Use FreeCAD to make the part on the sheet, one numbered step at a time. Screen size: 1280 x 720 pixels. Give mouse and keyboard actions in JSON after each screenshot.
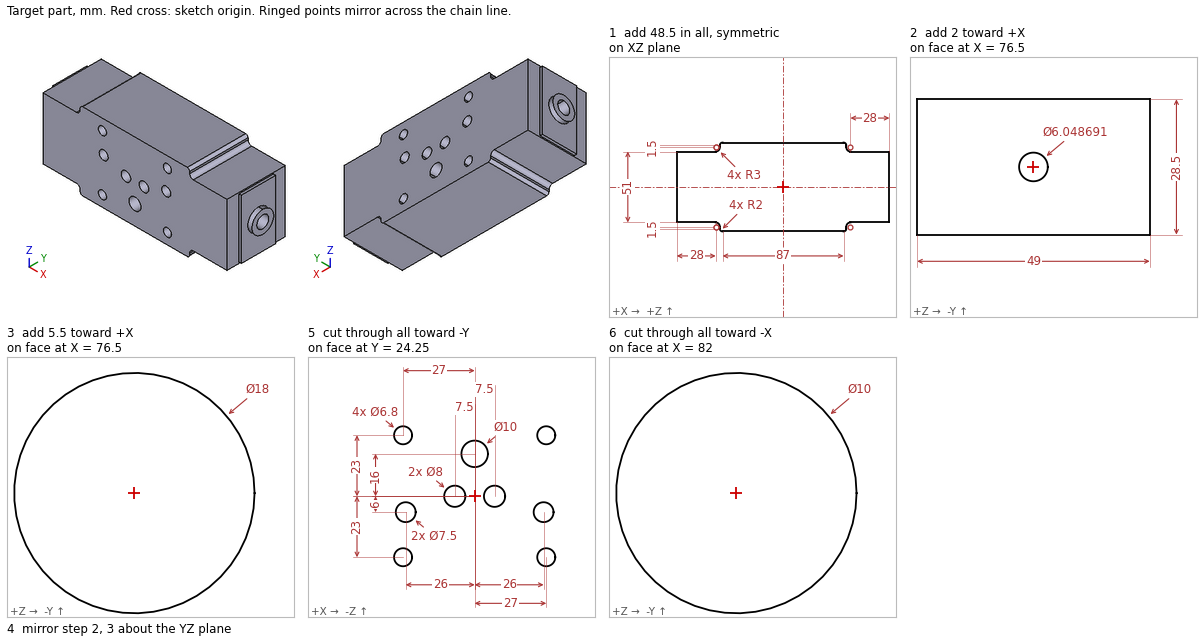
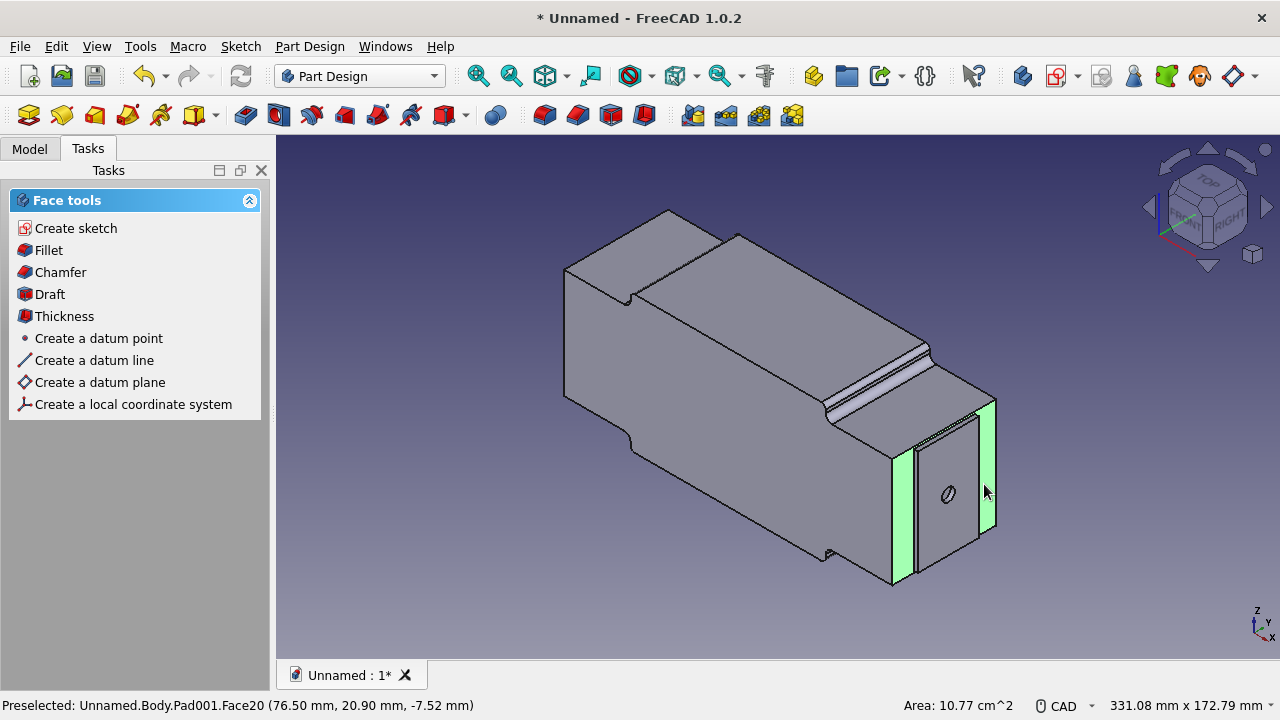
{"action": "left_click", "coordinate": [1056, 76]}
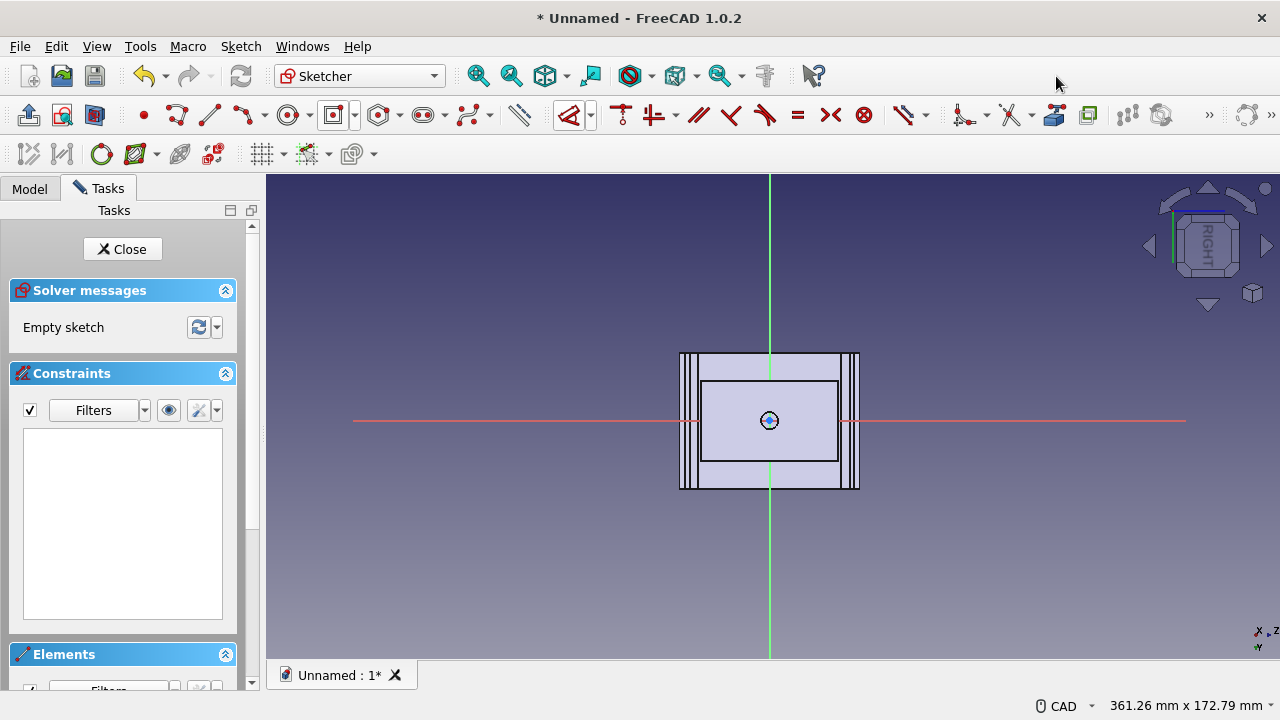
{"action": "key", "text": "q s"}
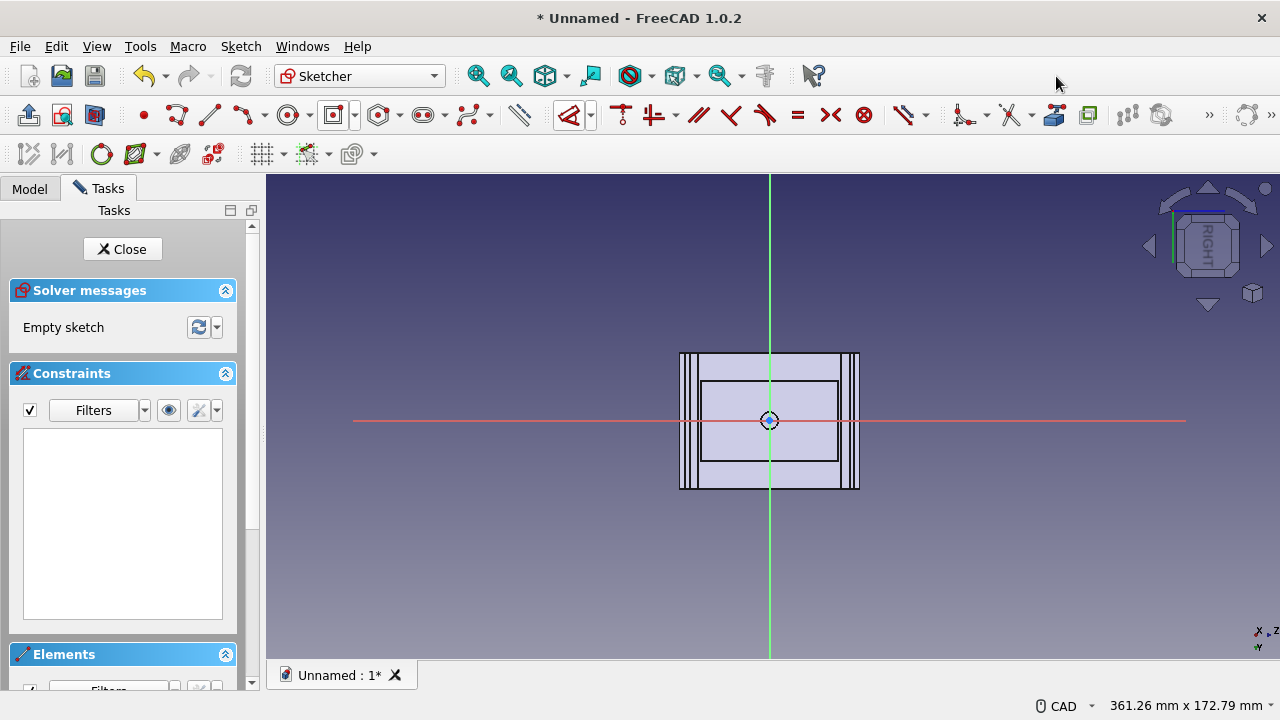
{"action": "scroll", "coordinate": [783, 421], "scroll_direction": "up", "scroll_amount": 9}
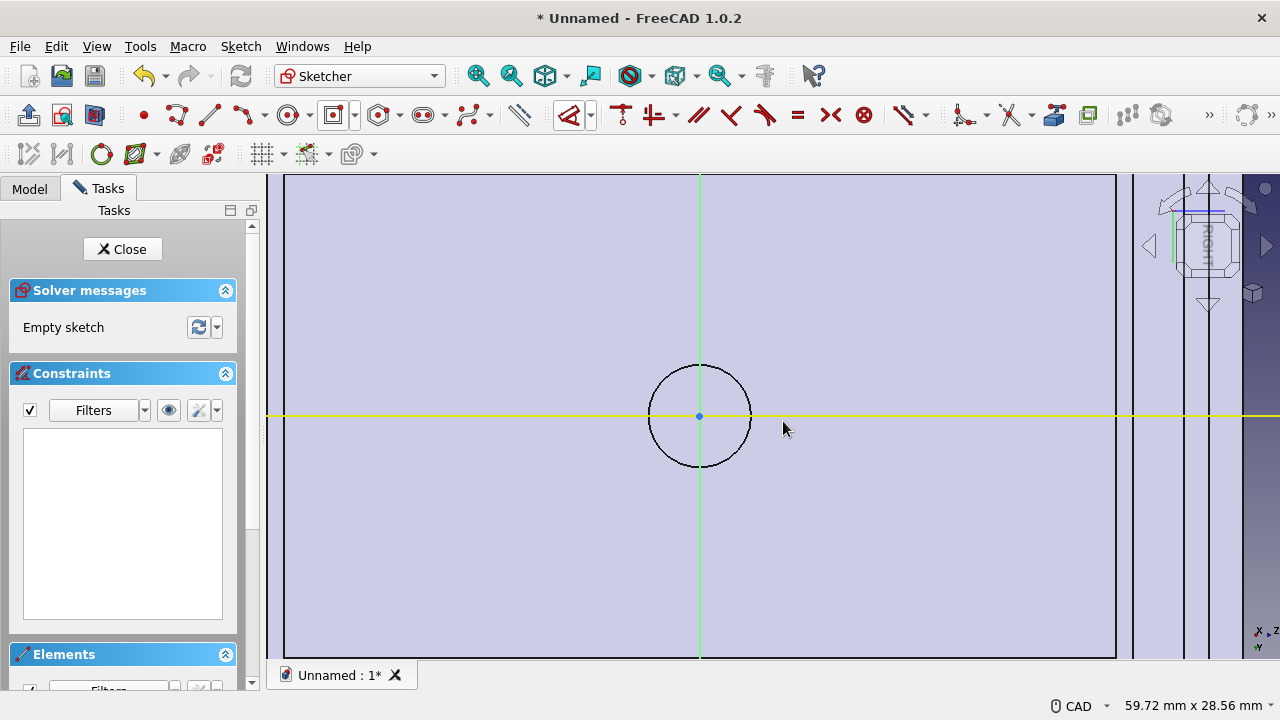
{"action": "left_click", "coordinate": [288, 116]}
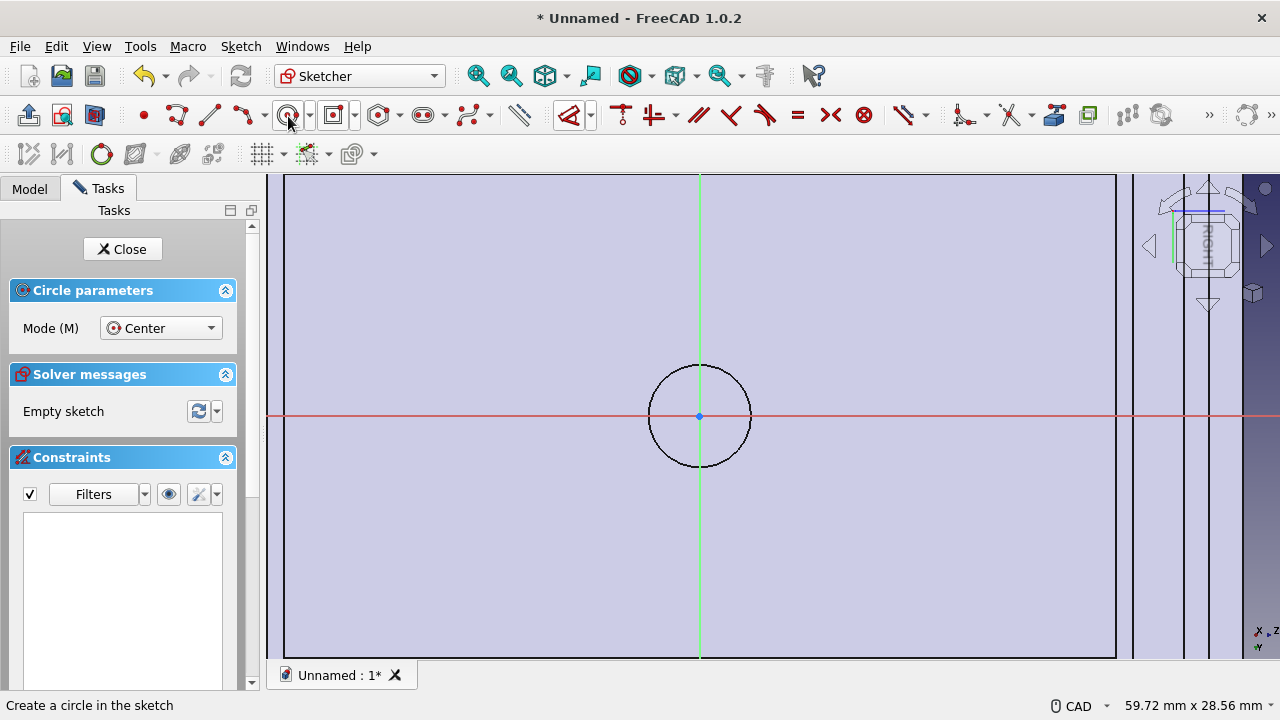
{"action": "left_click", "coordinate": [700, 416]}
{"action": "left_click", "coordinate": [808, 308]}
{"action": "key", "text": "Escape"}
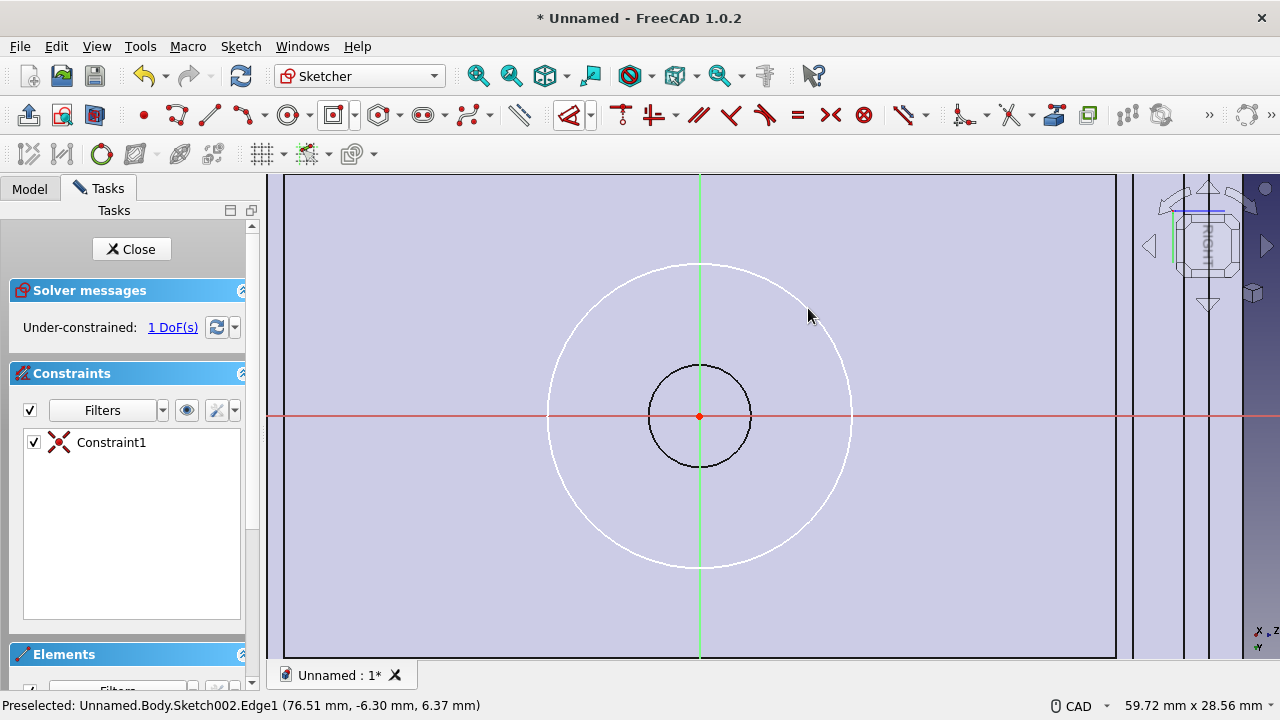
{"action": "left_click", "coordinate": [807, 308]}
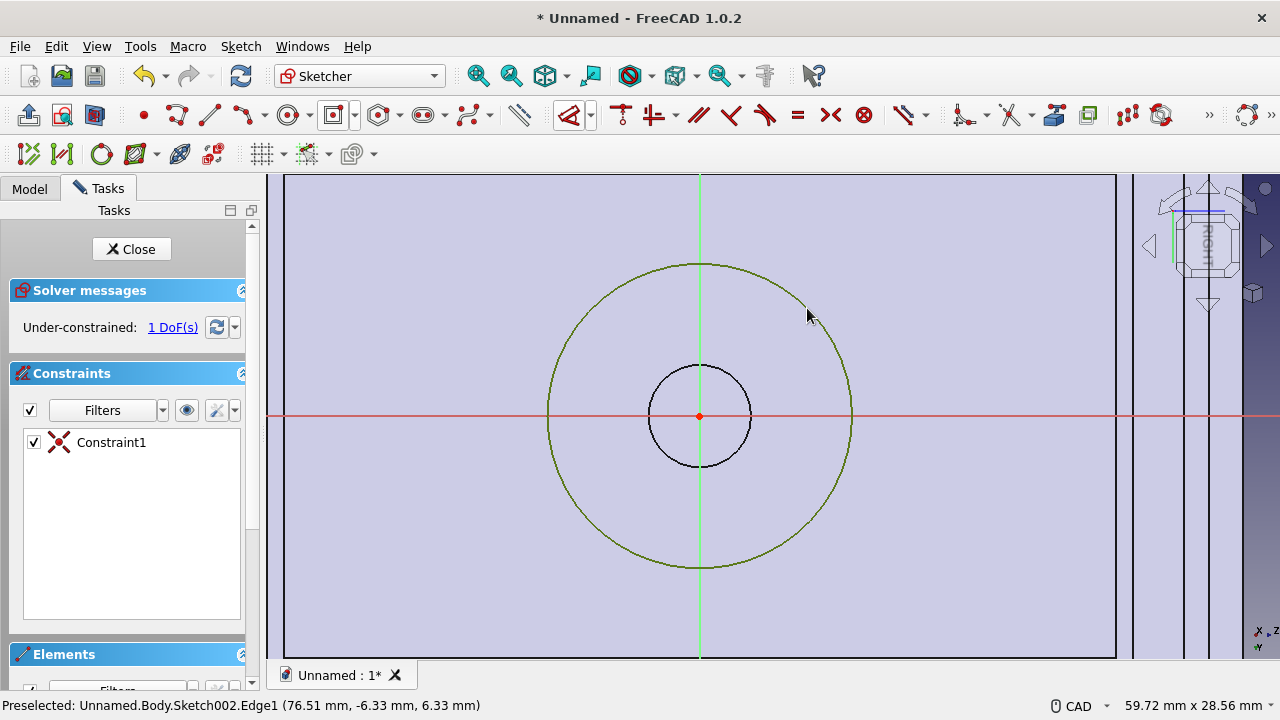
{"action": "key", "text": "k o"}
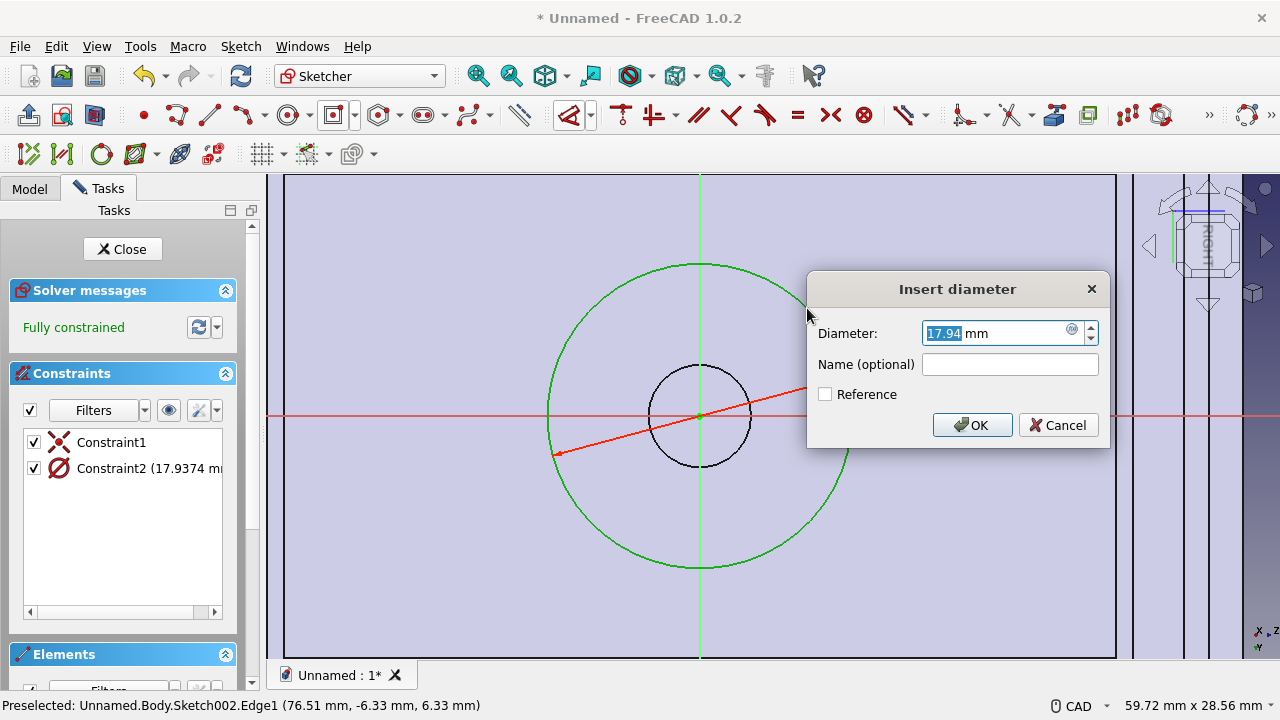
{"action": "type", "text": "18"}
{"action": "key", "text": "Return"}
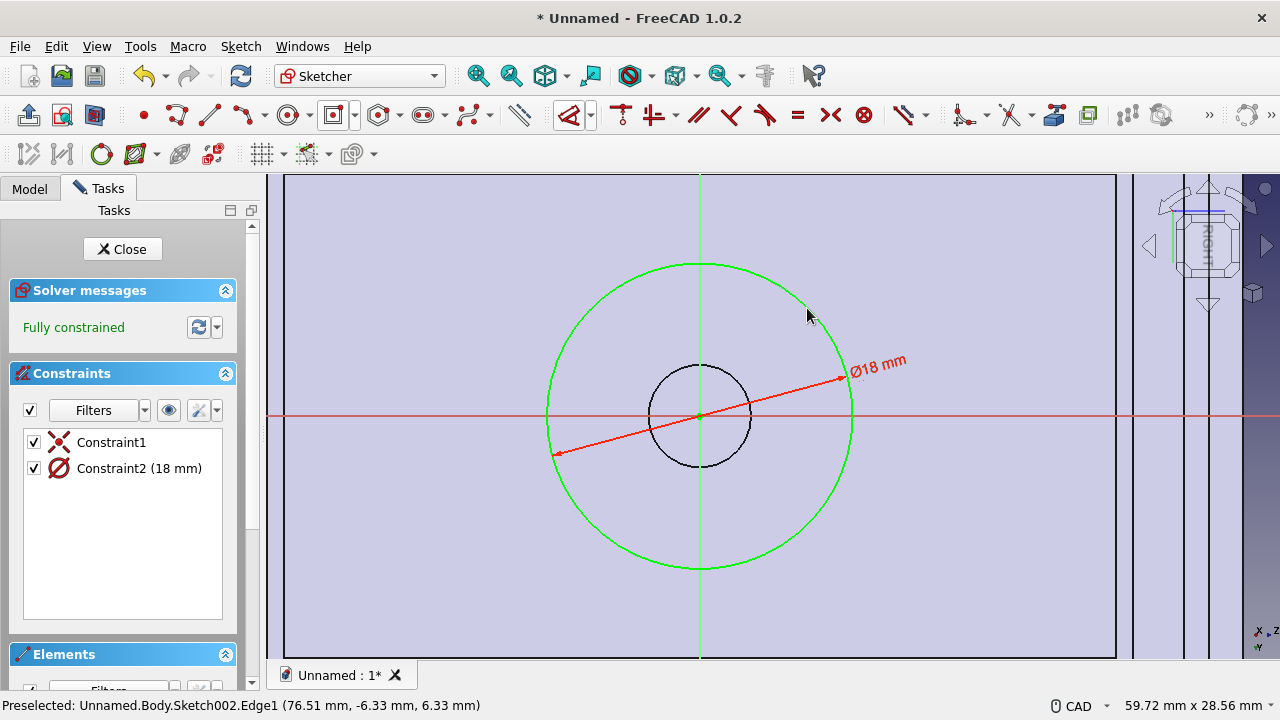
{"action": "left_click", "coordinate": [123, 249]}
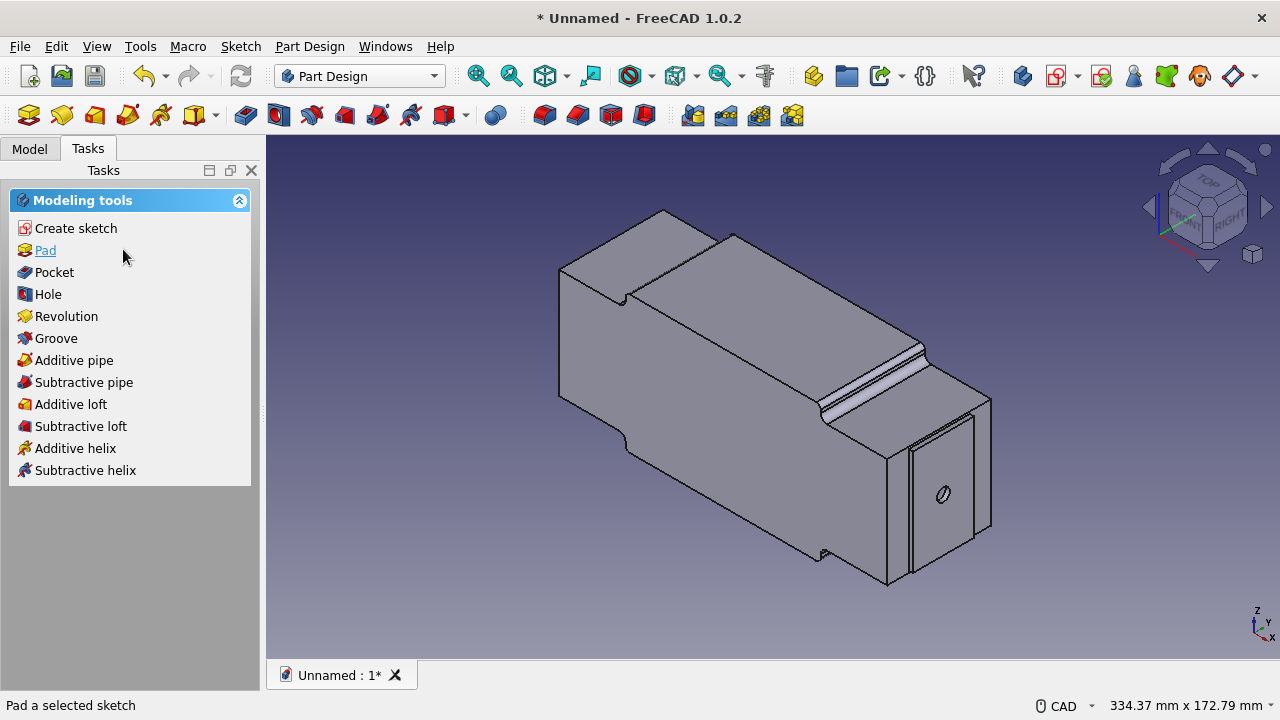
{"action": "left_click", "coordinate": [29, 116]}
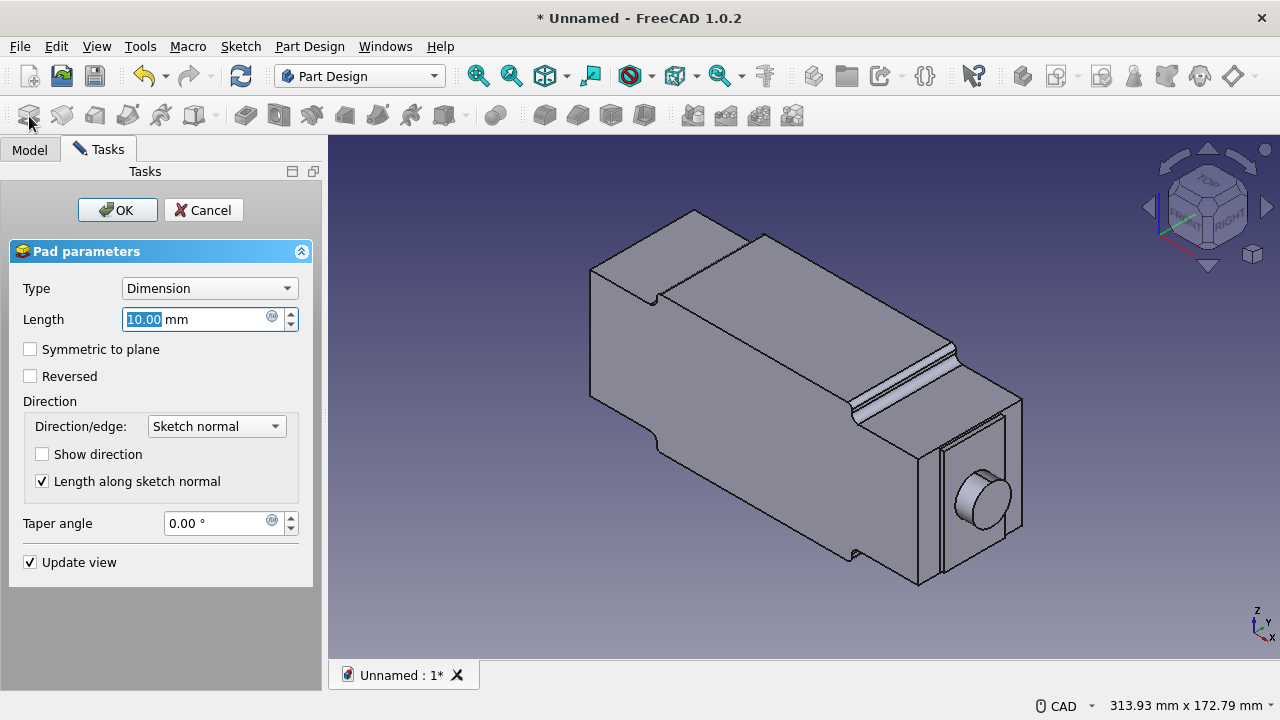
{"action": "type", "text": "5.5"}
{"action": "key", "text": "Tab"}